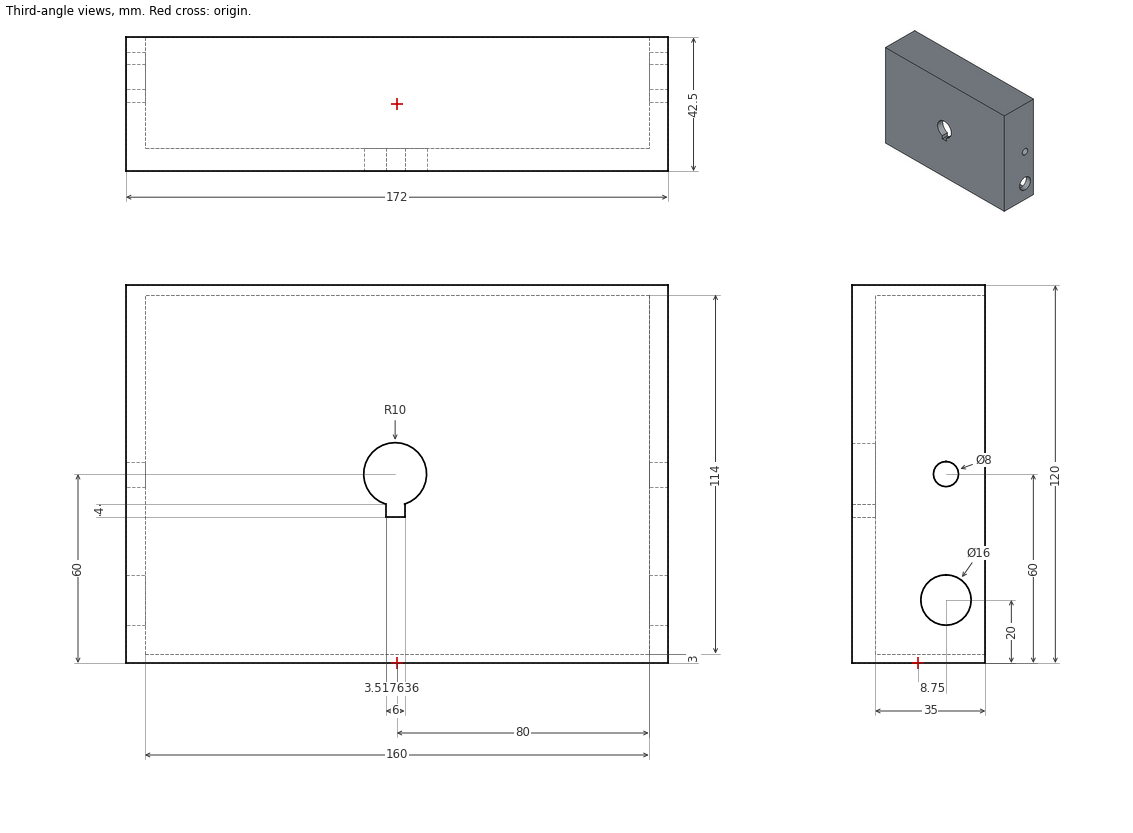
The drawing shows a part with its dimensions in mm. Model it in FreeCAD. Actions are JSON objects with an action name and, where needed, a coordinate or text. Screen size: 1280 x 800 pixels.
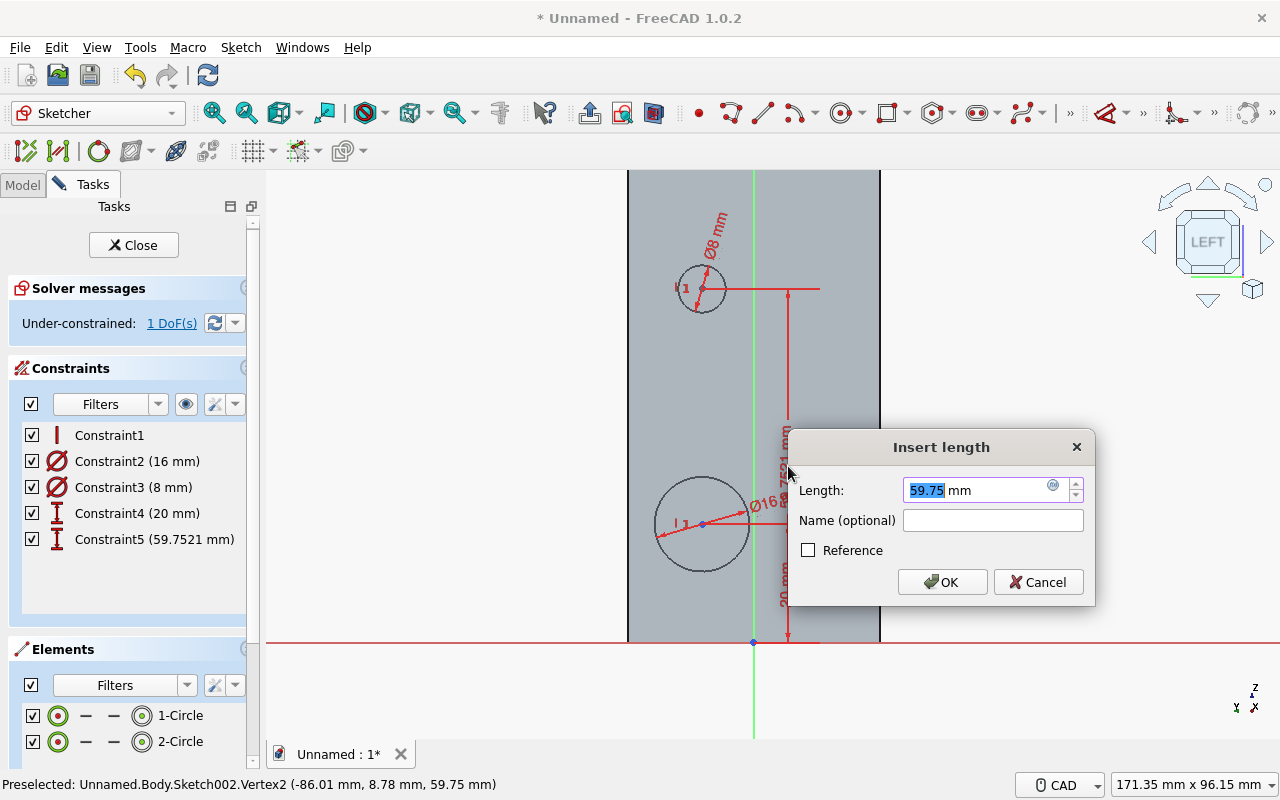
{"action": "type", "text": "60"}
{"action": "key", "text": "Return"}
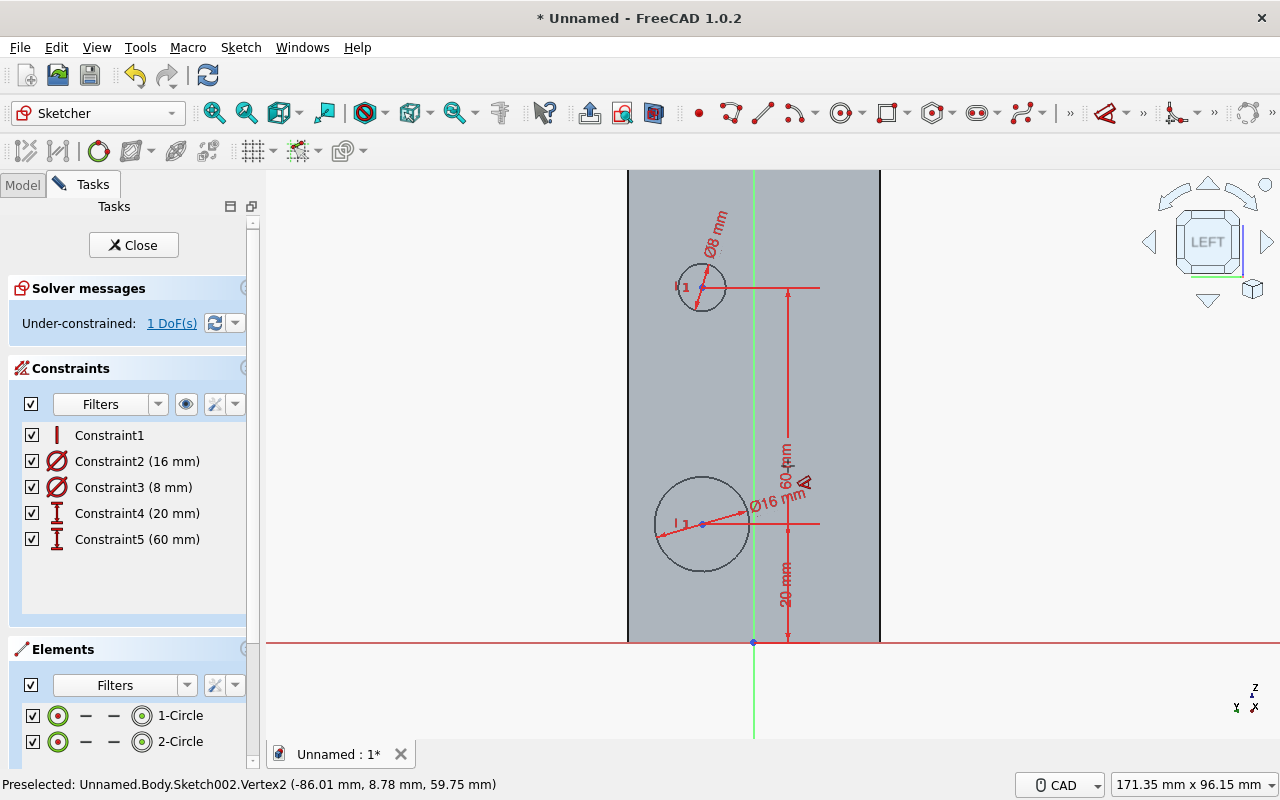
{"action": "left_click", "coordinate": [702, 524]}
{"action": "left_click", "coordinate": [728, 677]}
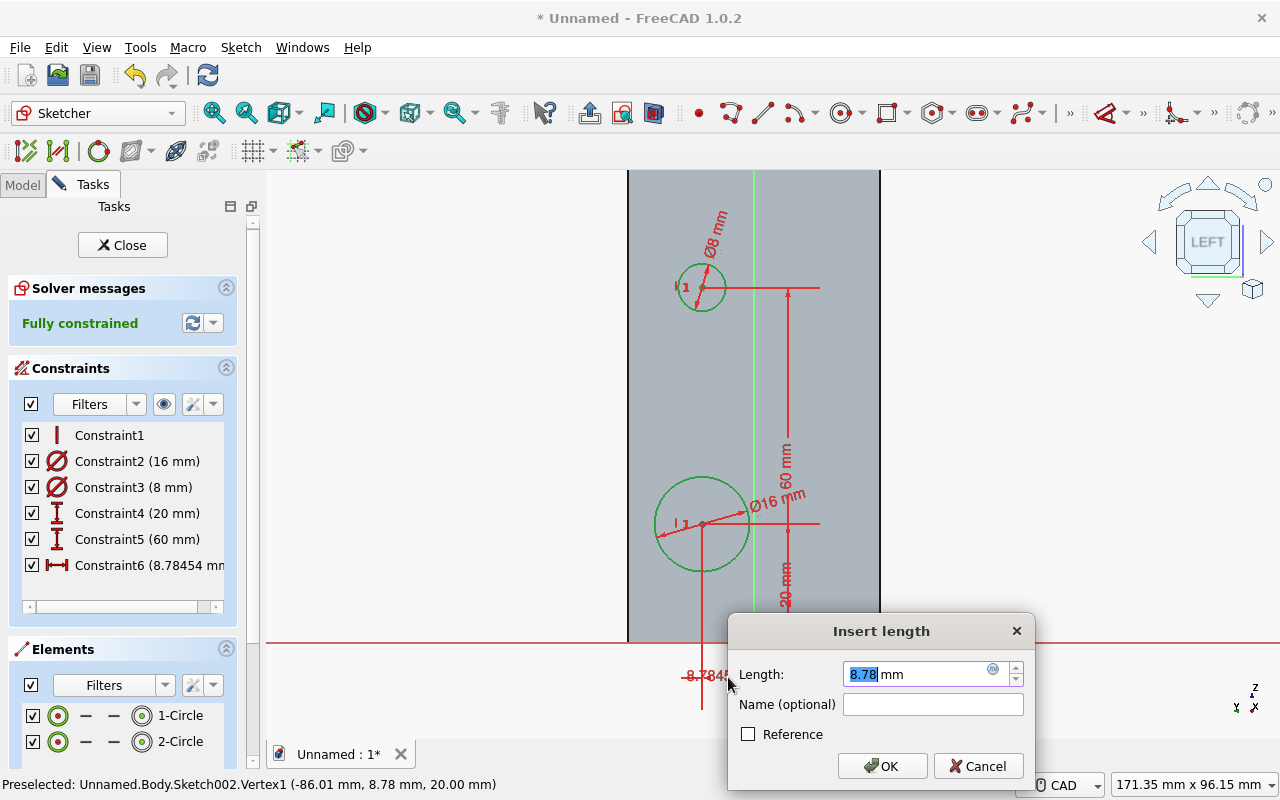
{"action": "type", "text": "8.75"}
{"action": "key", "text": "Return"}
{"action": "key", "text": "Escape"}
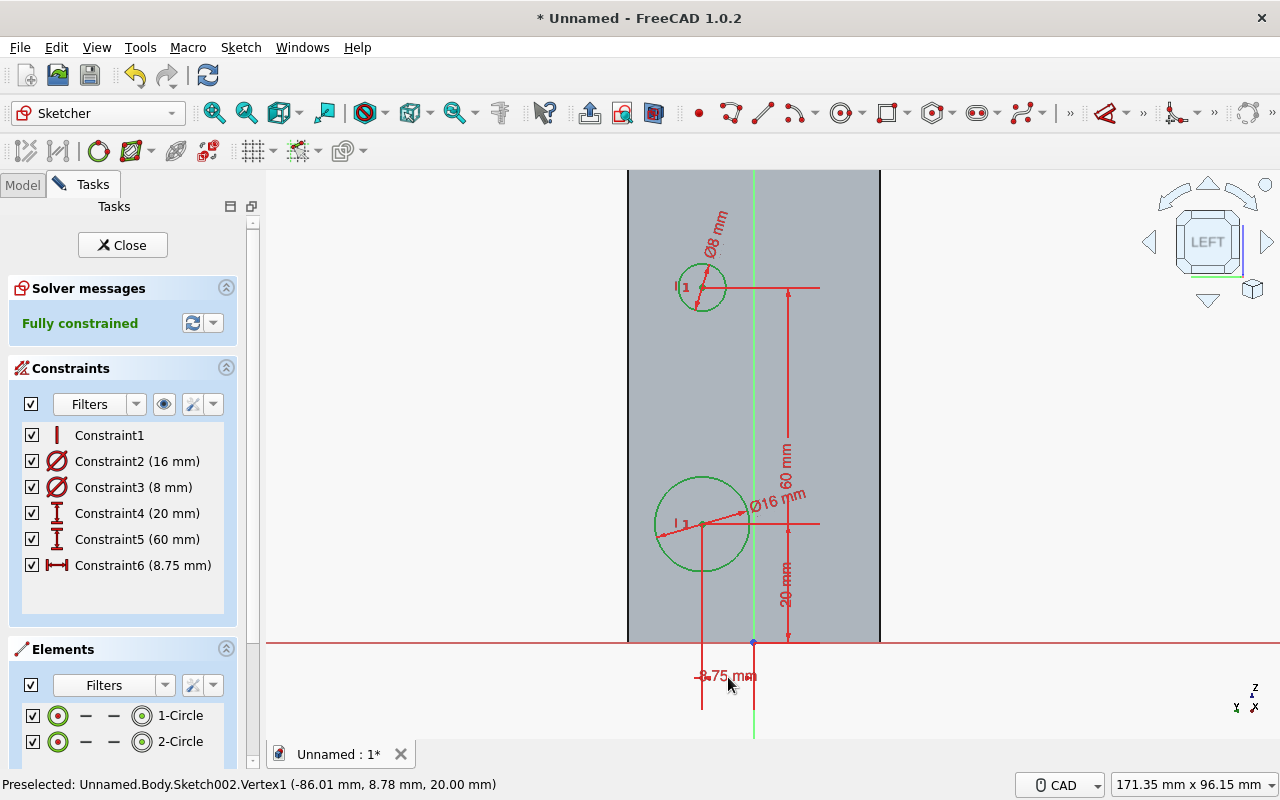
{"action": "left_click", "coordinate": [123, 245]}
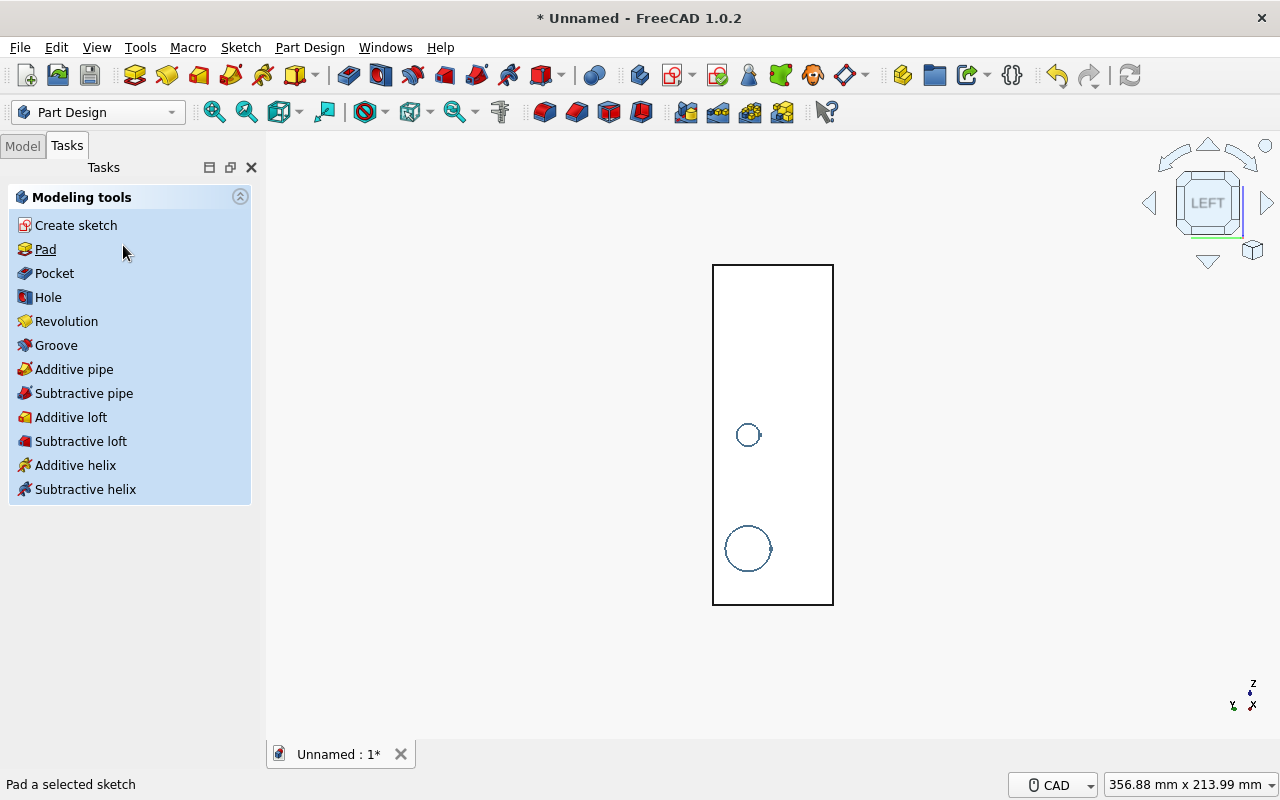
{"action": "left_click", "coordinate": [350, 76]}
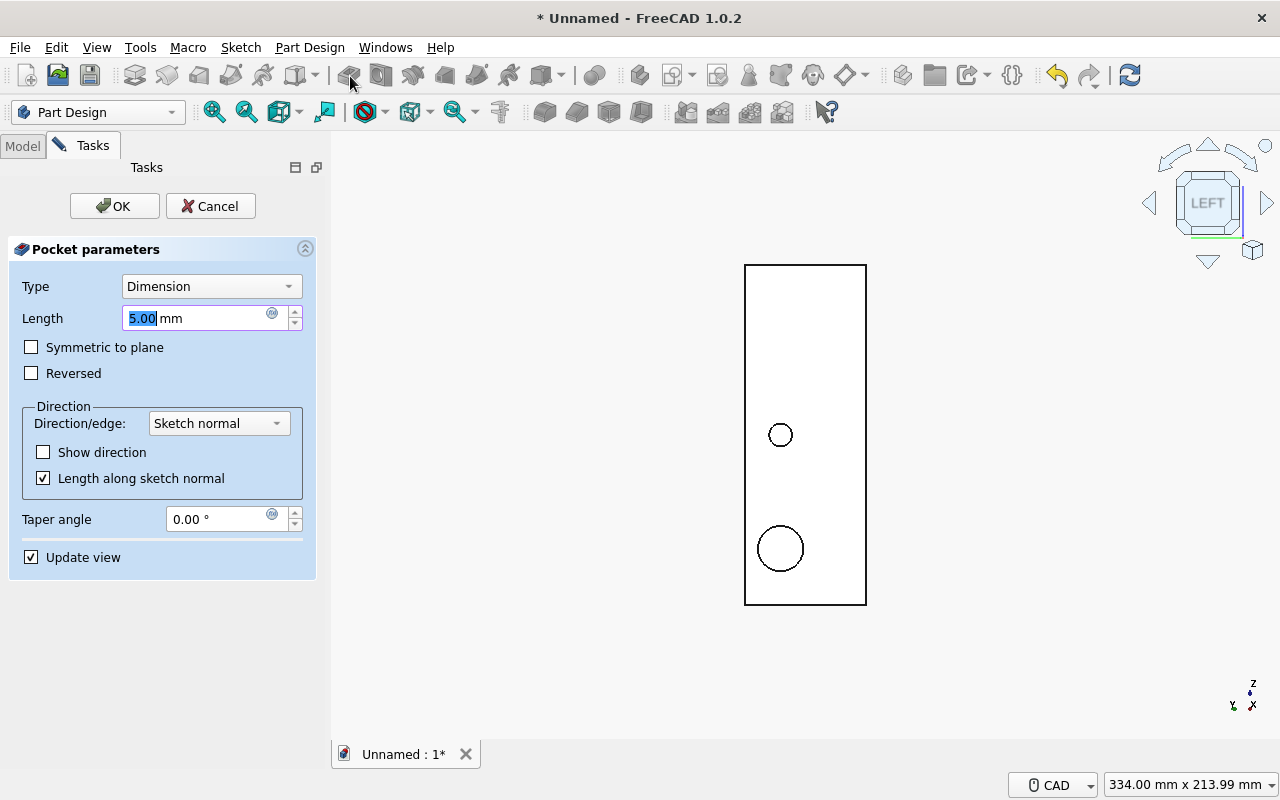
{"action": "left_click", "coordinate": [212, 286]}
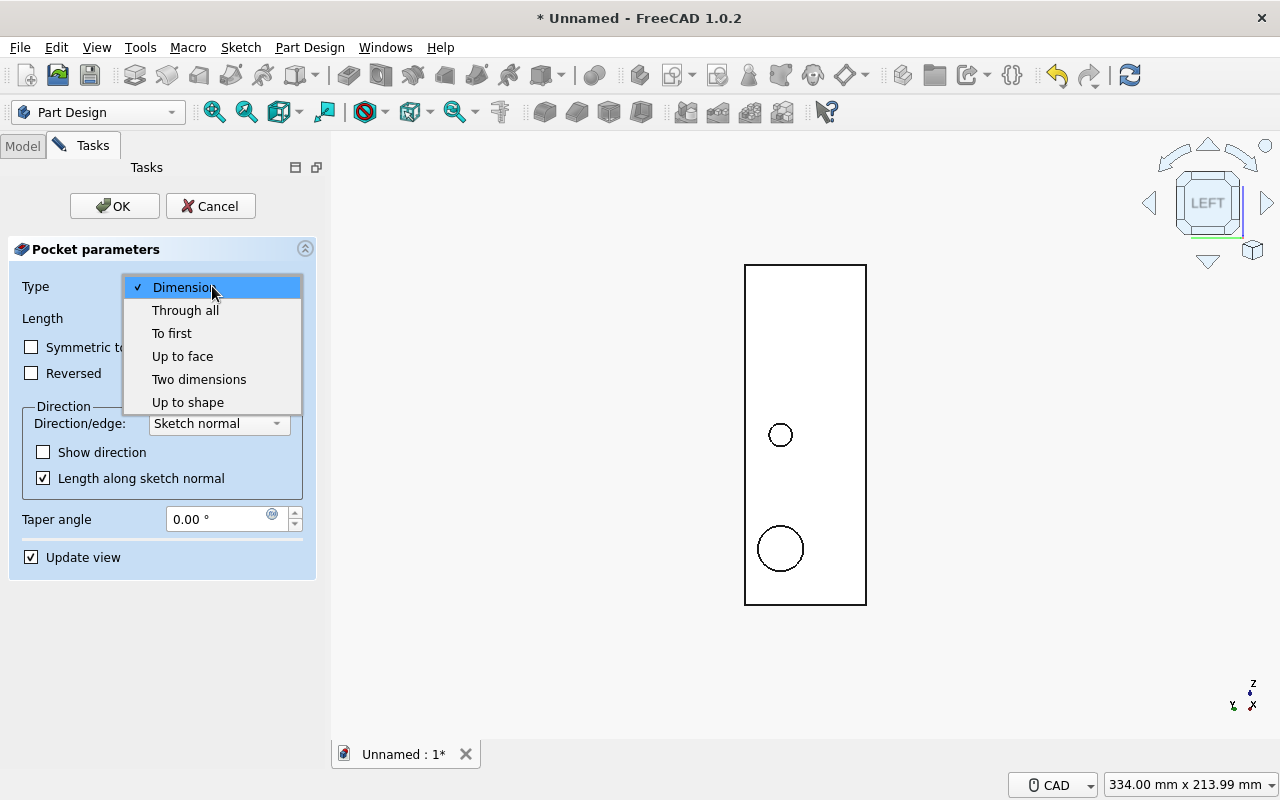
{"action": "left_click", "coordinate": [212, 310]}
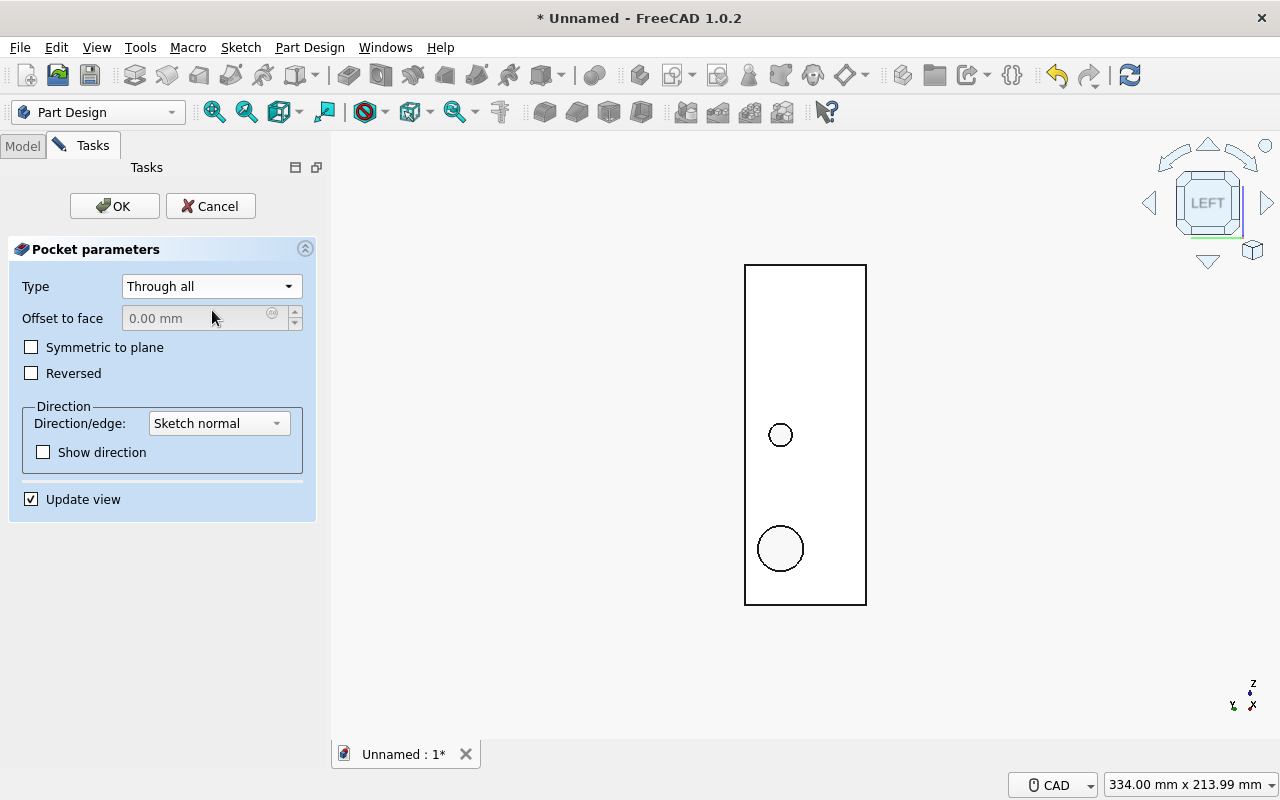
{"action": "left_click", "coordinate": [115, 206]}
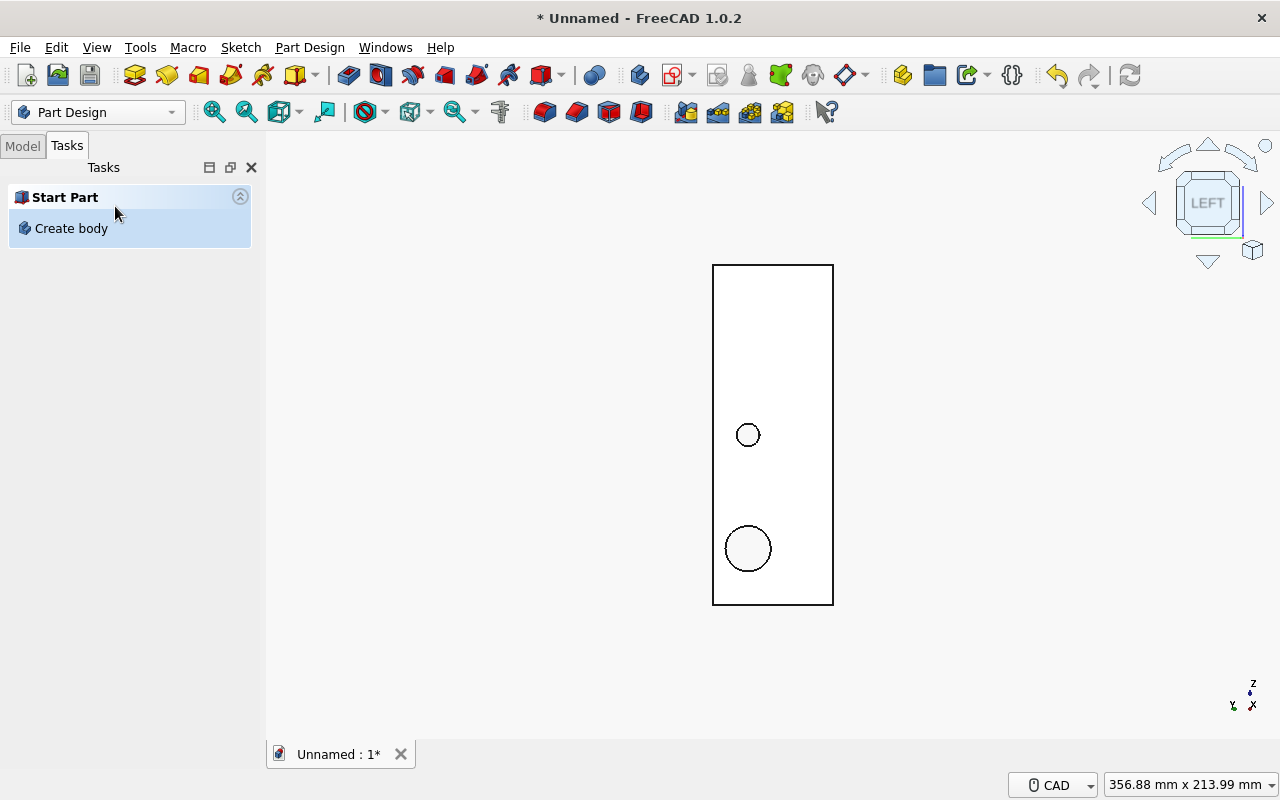
{"action": "key", "text": "0"}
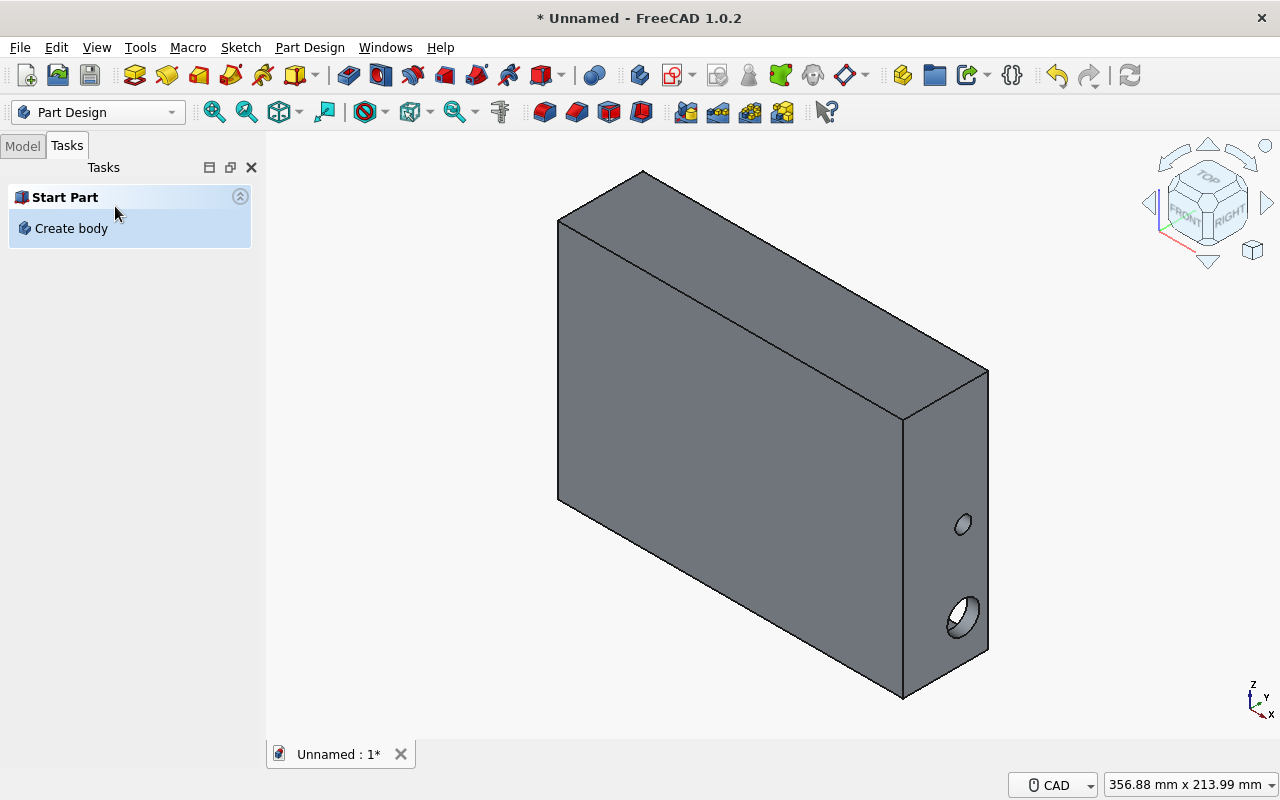
{"action": "left_click", "coordinate": [780, 487]}